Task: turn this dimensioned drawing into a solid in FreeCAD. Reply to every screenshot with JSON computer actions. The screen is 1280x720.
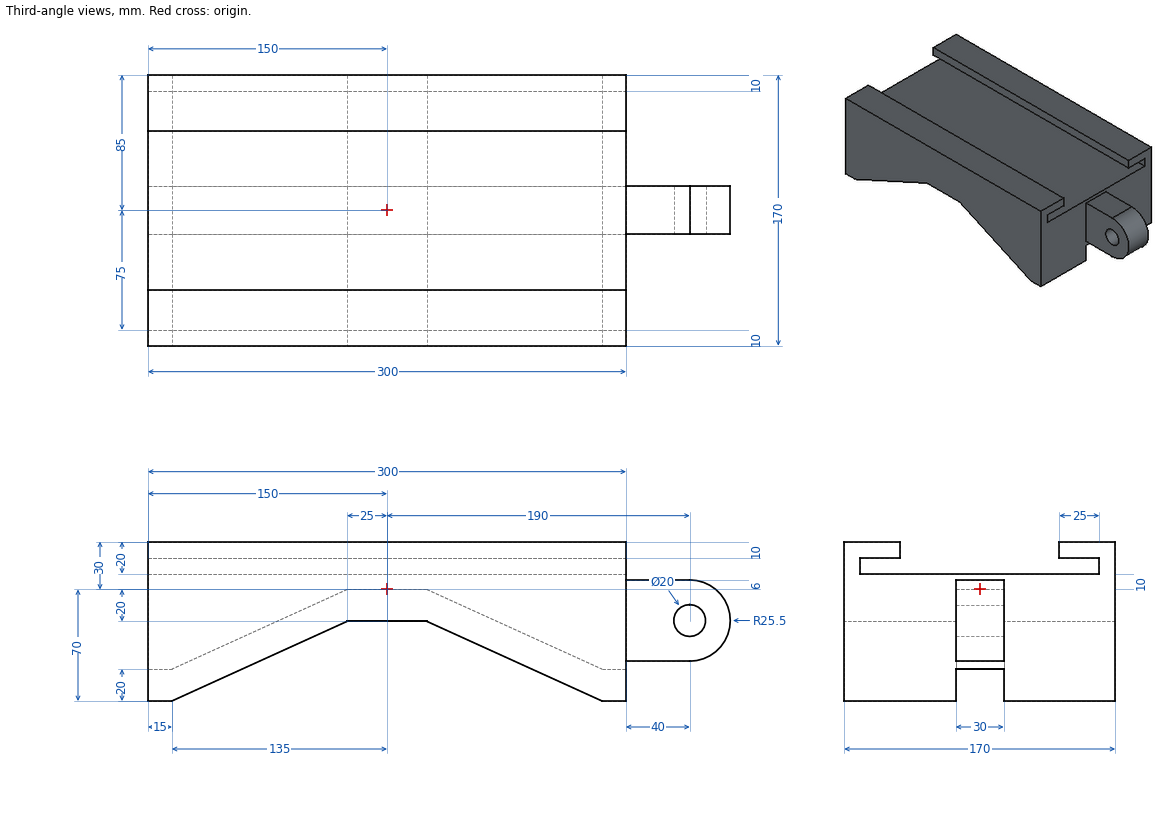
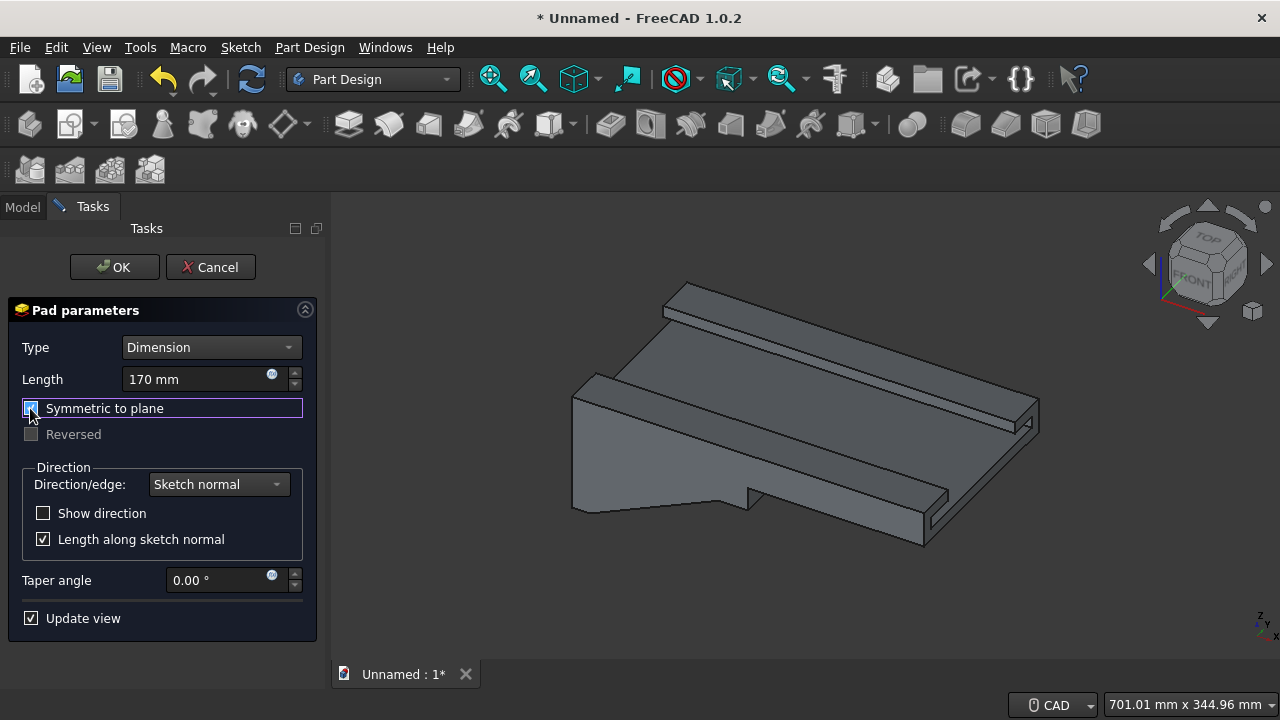
{"action": "left_click", "coordinate": [115, 267]}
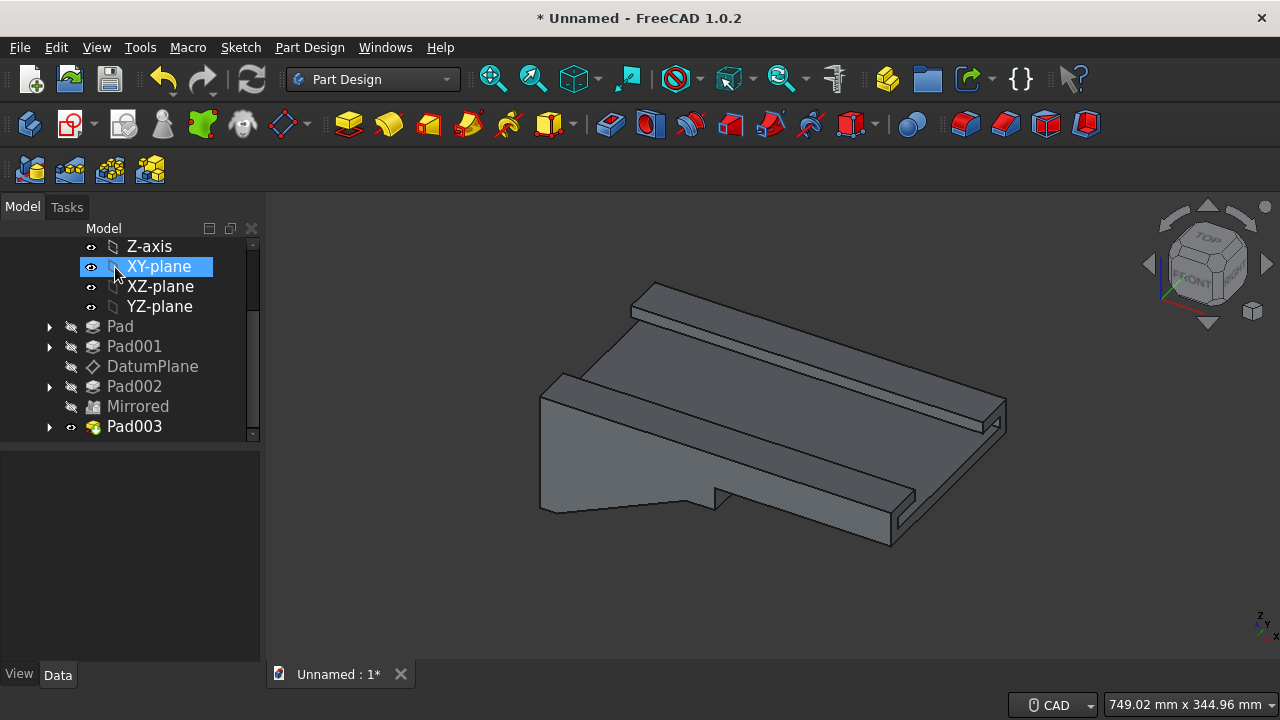
{"action": "left_click", "coordinate": [70, 124]}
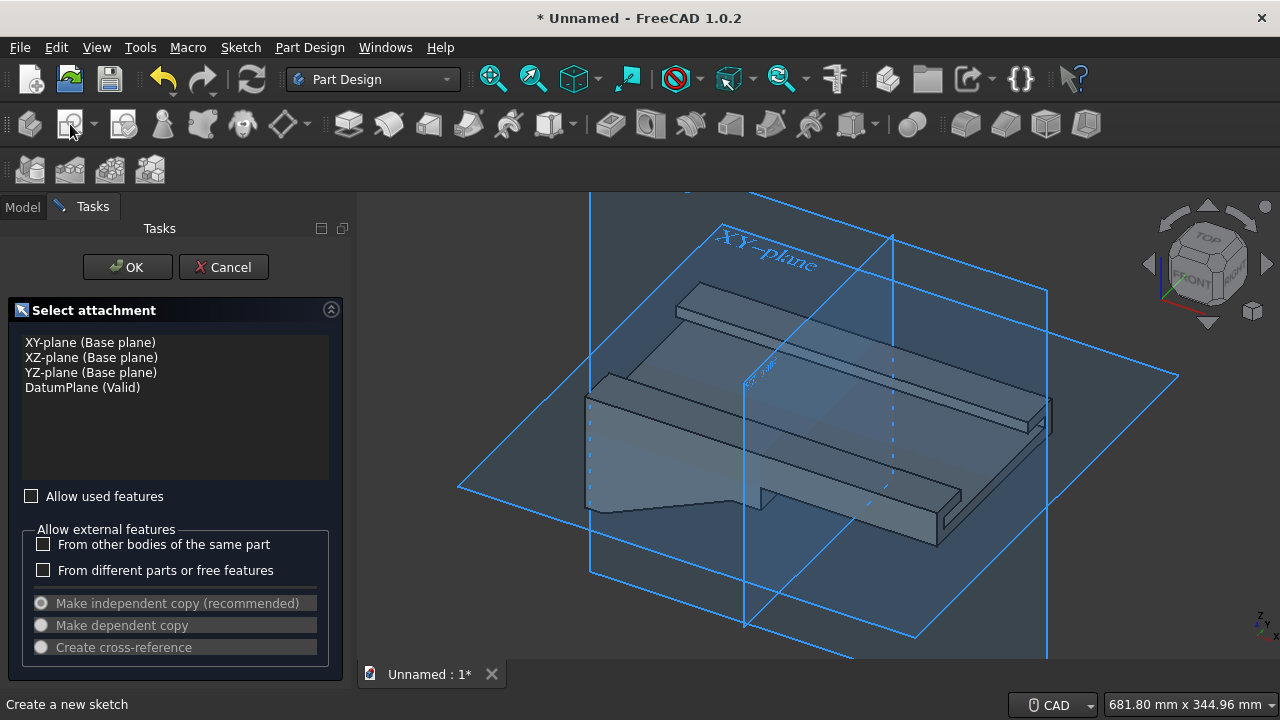
{"action": "left_click", "coordinate": [82, 358]}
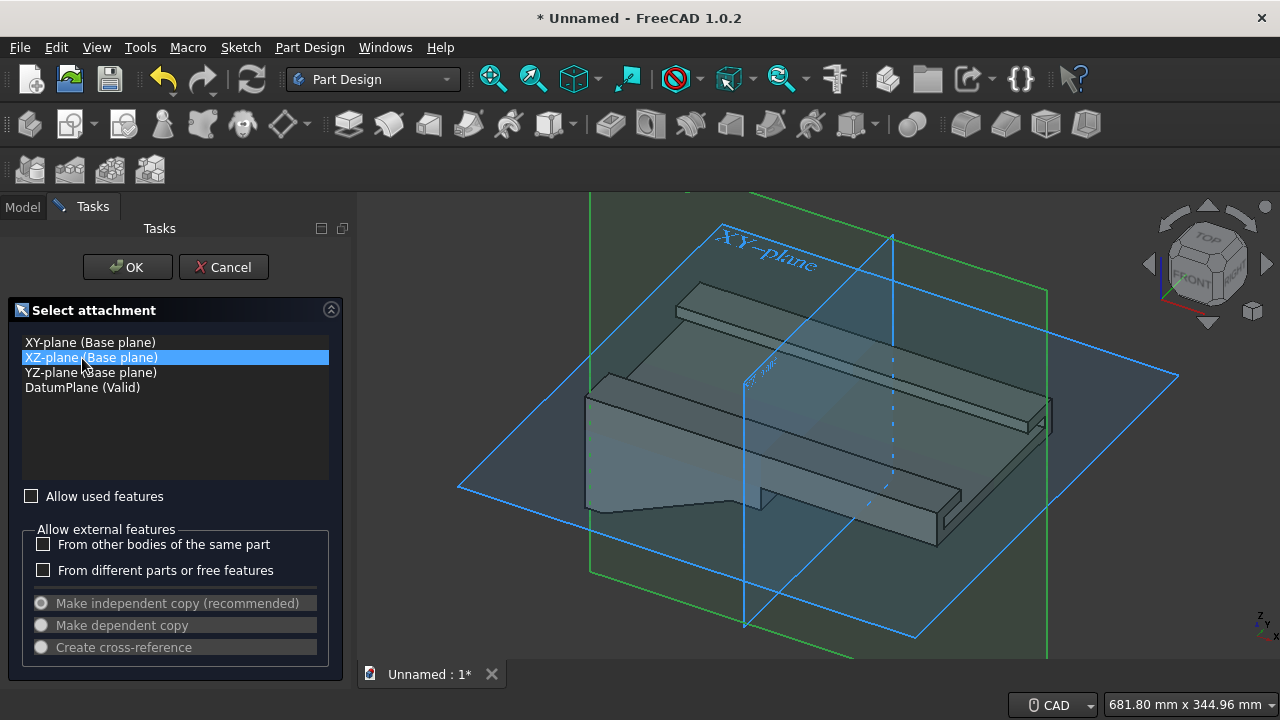
{"action": "left_click", "coordinate": [128, 267]}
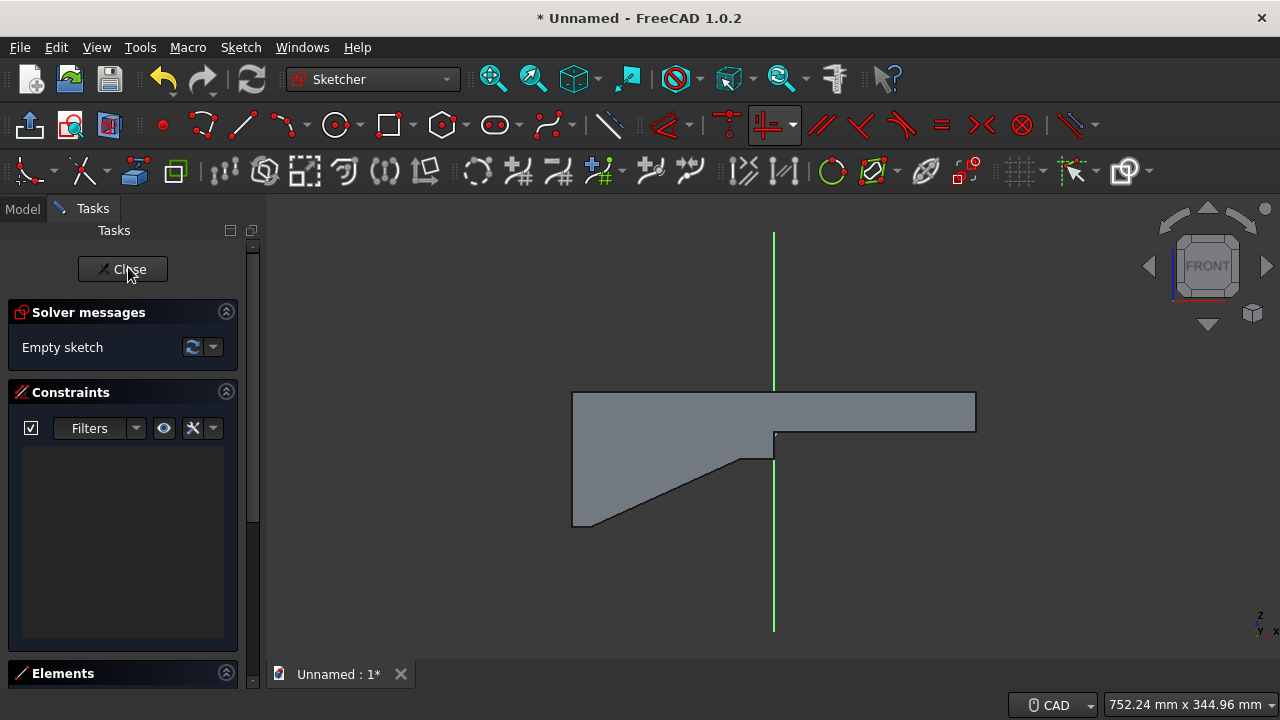
{"action": "key", "text": "q s"}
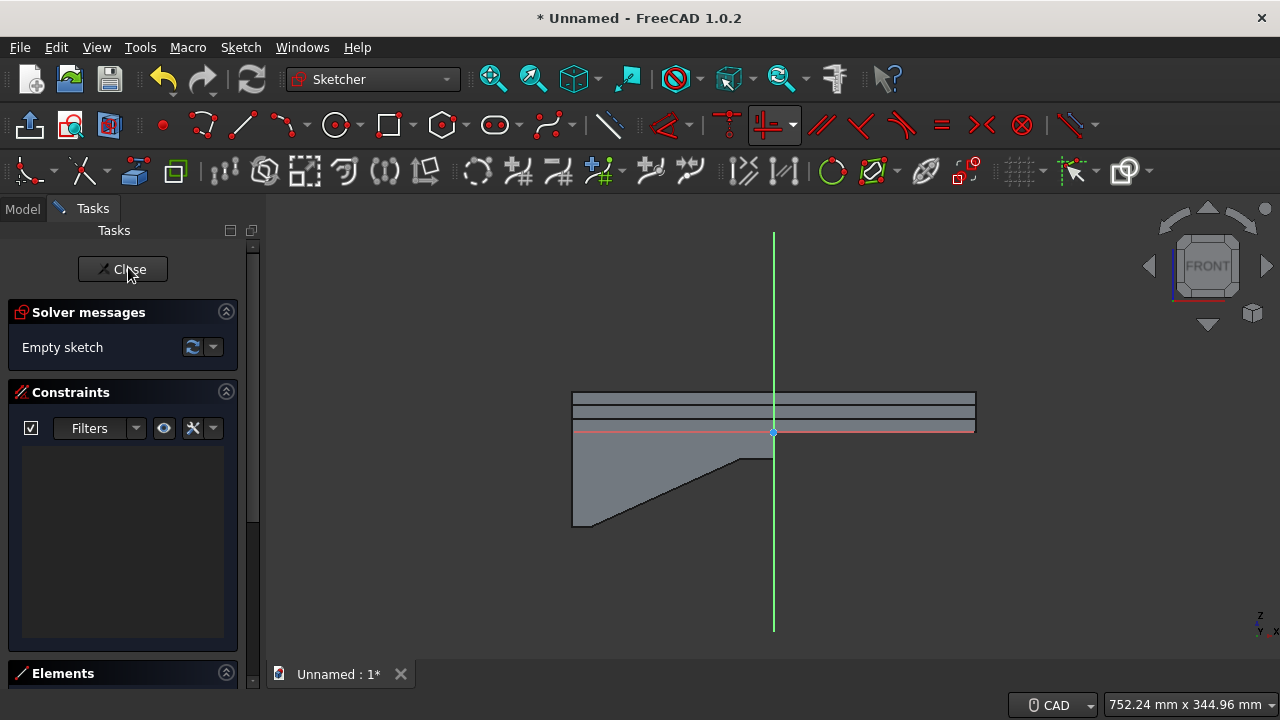
{"action": "scroll", "coordinate": [654, 510], "scroll_direction": "up", "scroll_amount": 5}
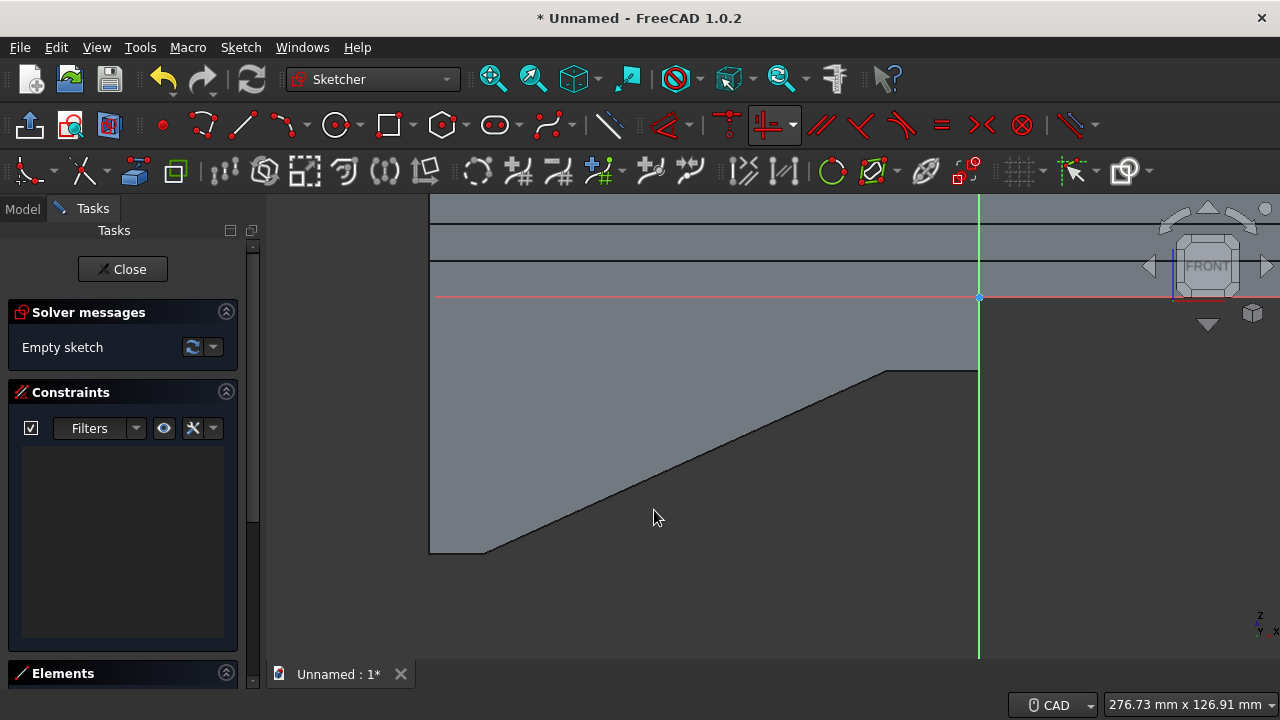
{"action": "key", "text": "g m"}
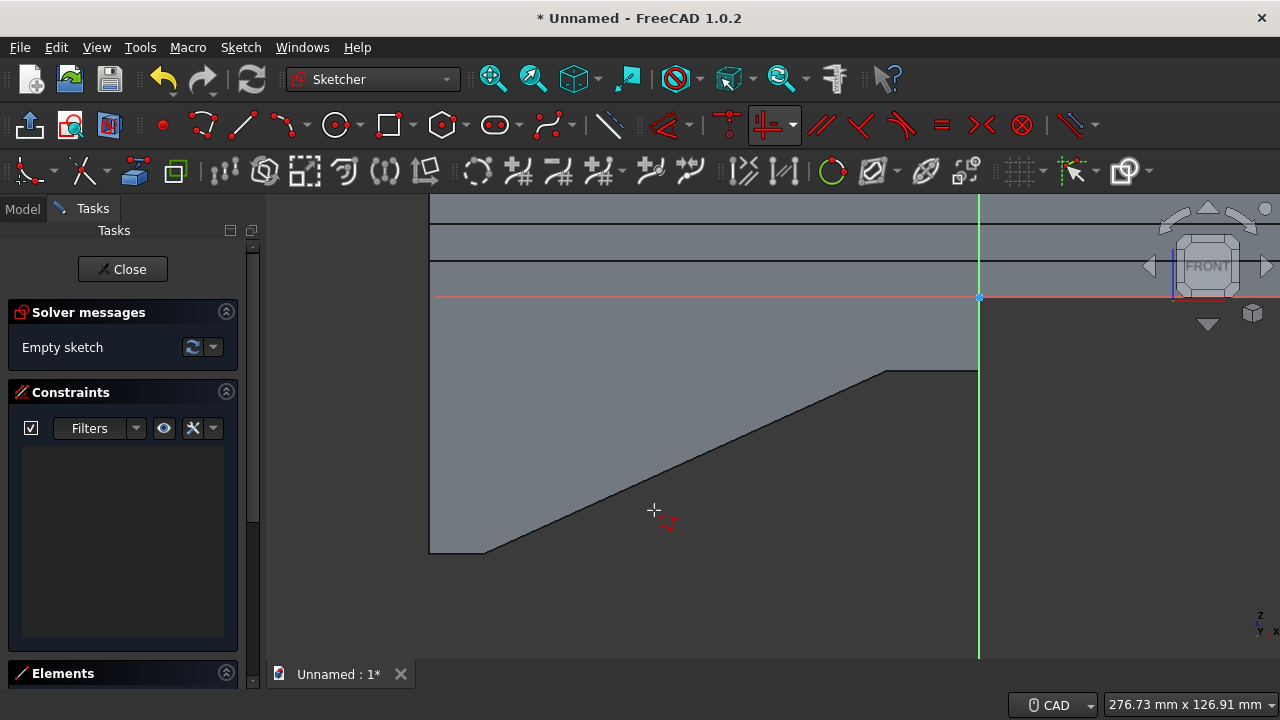
{"action": "left_click", "coordinate": [979, 297]}
{"action": "left_click", "coordinate": [970, 371]}
{"action": "left_click", "coordinate": [887, 371]}
{"action": "left_click", "coordinate": [484, 554]}
{"action": "left_click", "coordinate": [429, 554]}
{"action": "left_click", "coordinate": [429, 480]}
{"action": "left_click", "coordinate": [484, 480]}
{"action": "left_click", "coordinate": [887, 306]}
{"action": "left_click", "coordinate": [979, 297]}
{"action": "key", "text": "Escape"}
{"action": "key", "text": "Escape"}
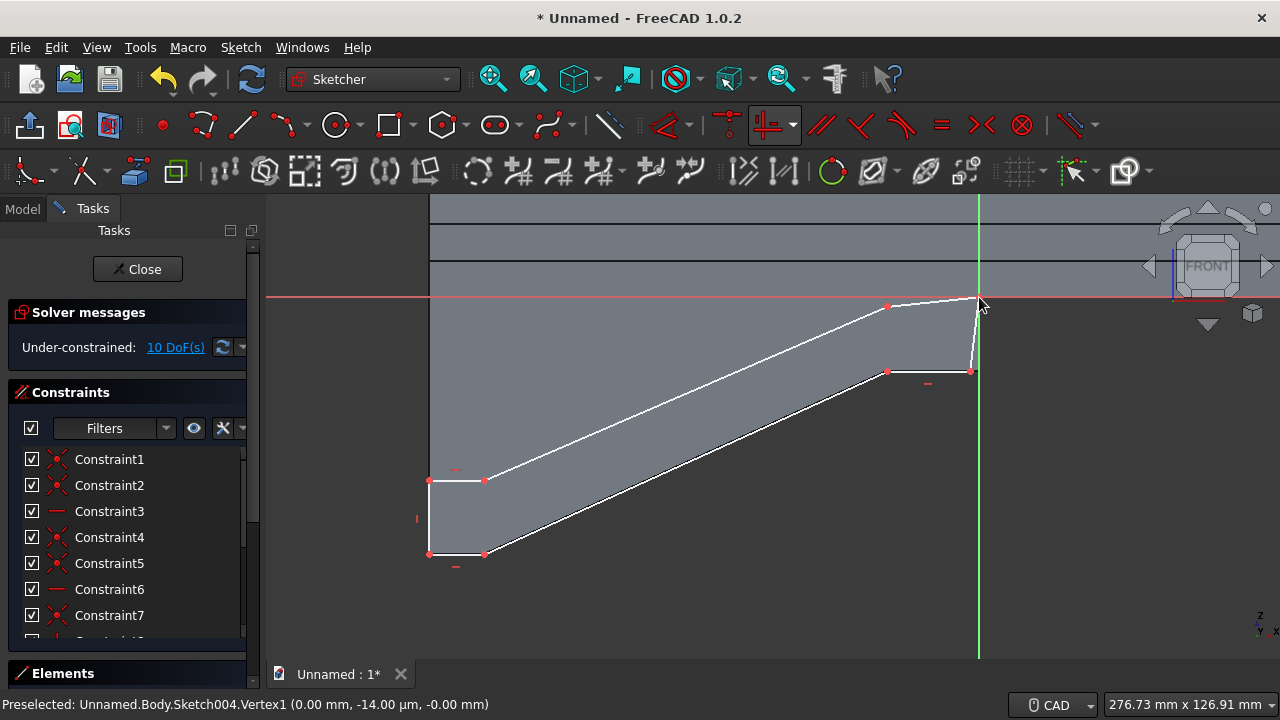
{"action": "left_click", "coordinate": [976, 320]}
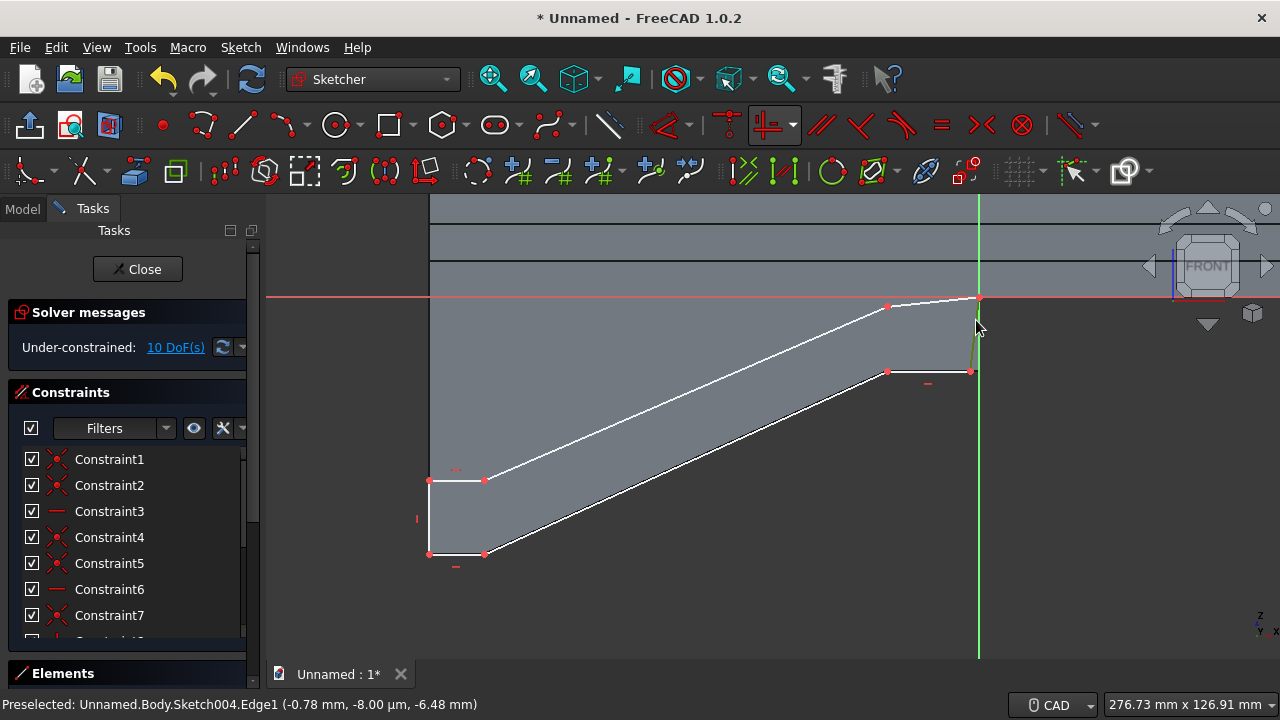
{"action": "left_click", "coordinate": [796, 126]}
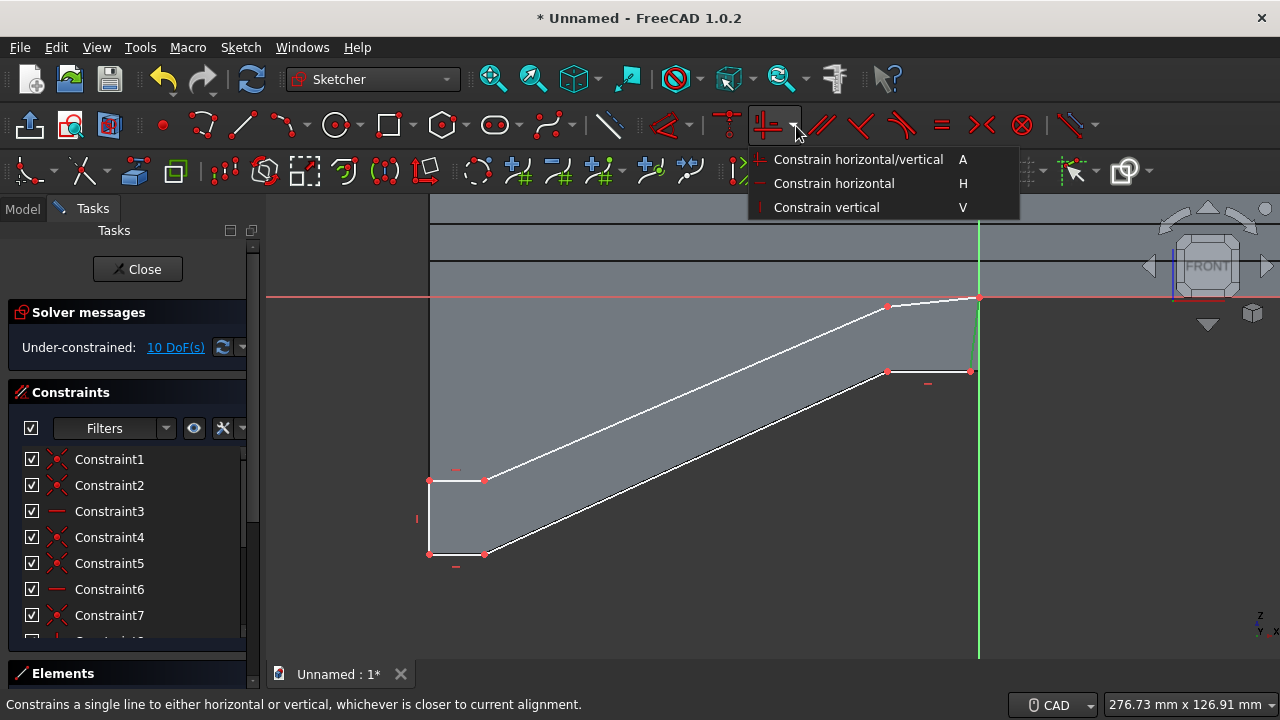
{"action": "left_click", "coordinate": [884, 207]}